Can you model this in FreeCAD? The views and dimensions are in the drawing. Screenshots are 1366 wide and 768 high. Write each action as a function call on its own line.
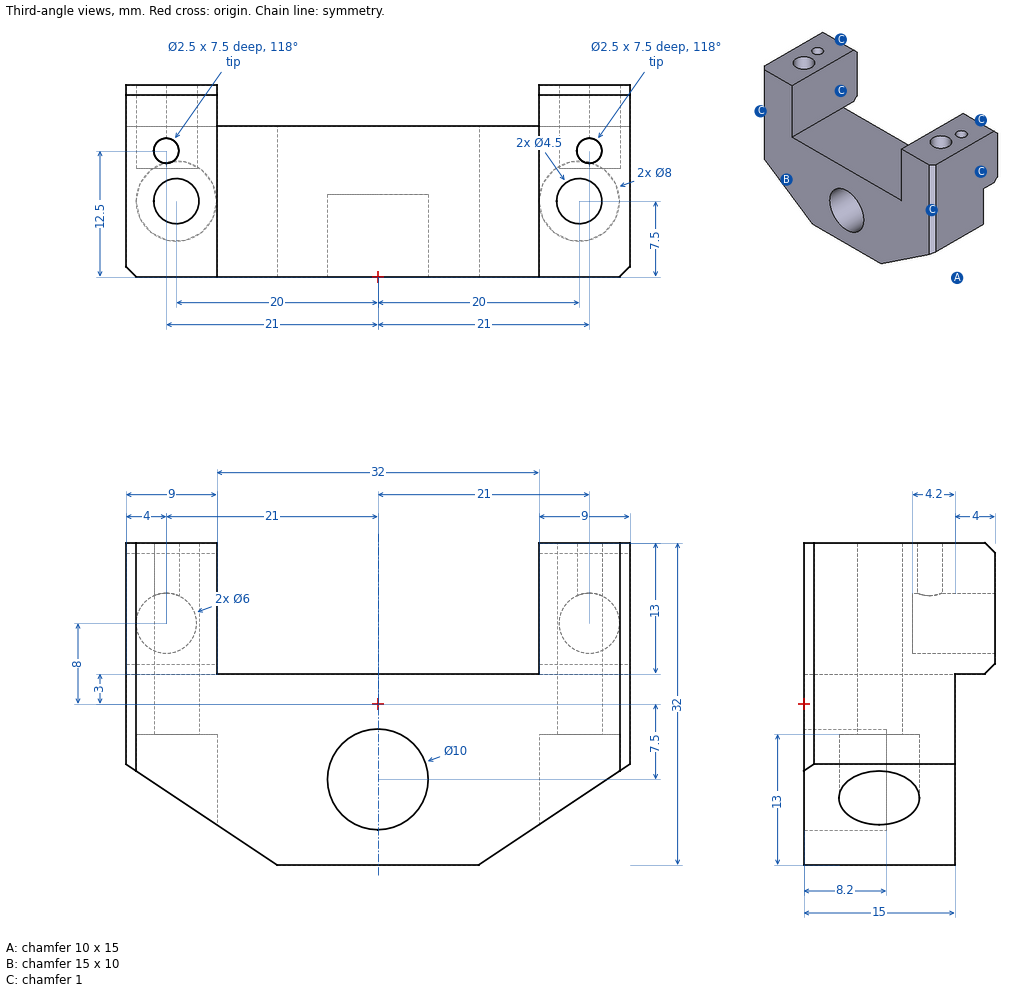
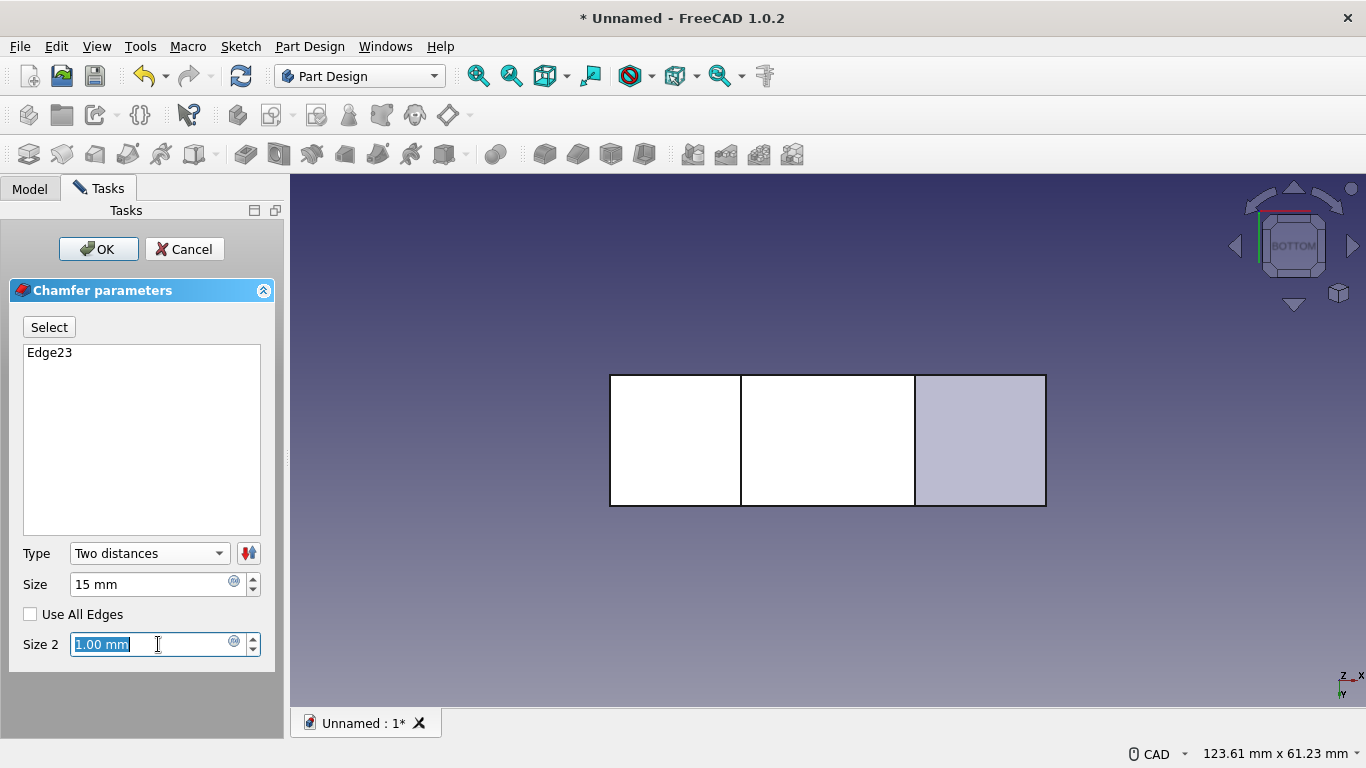
text(10)
key(Tab)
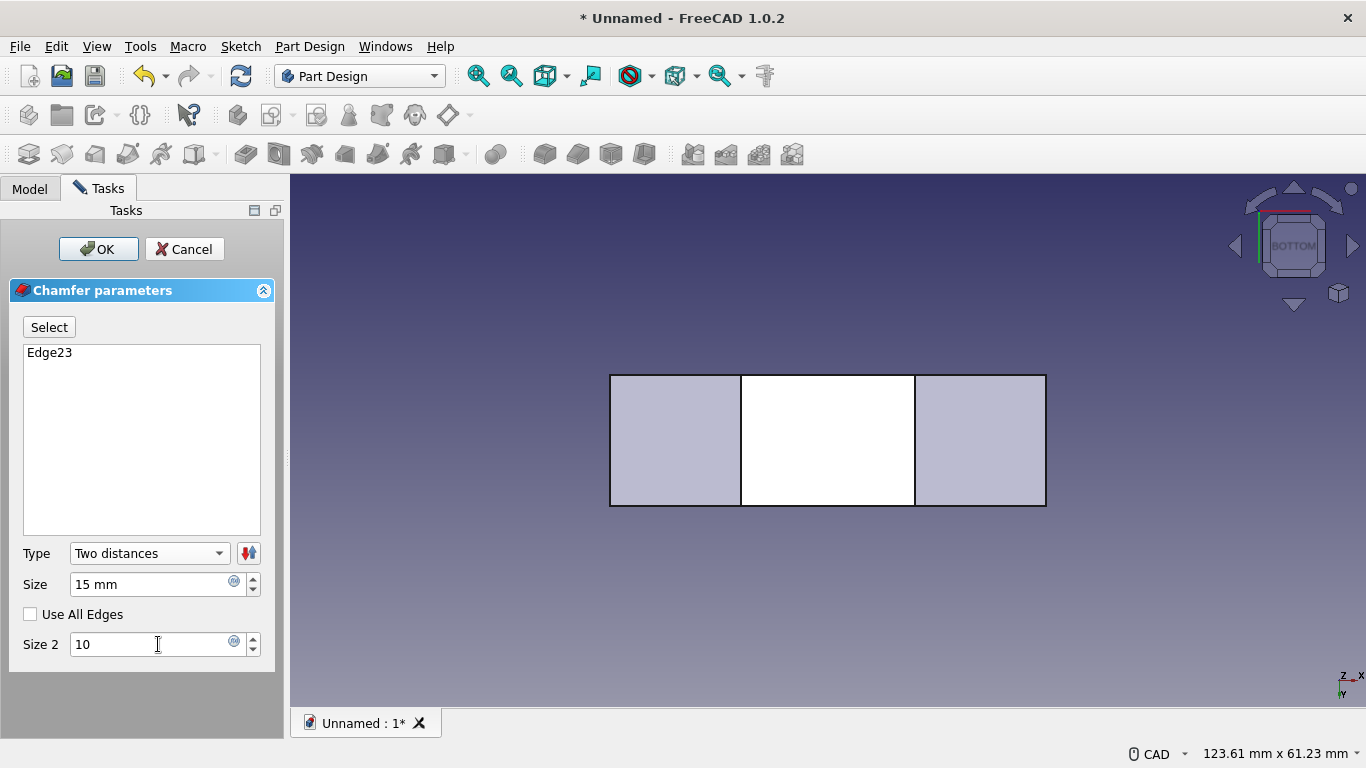
click(99, 249)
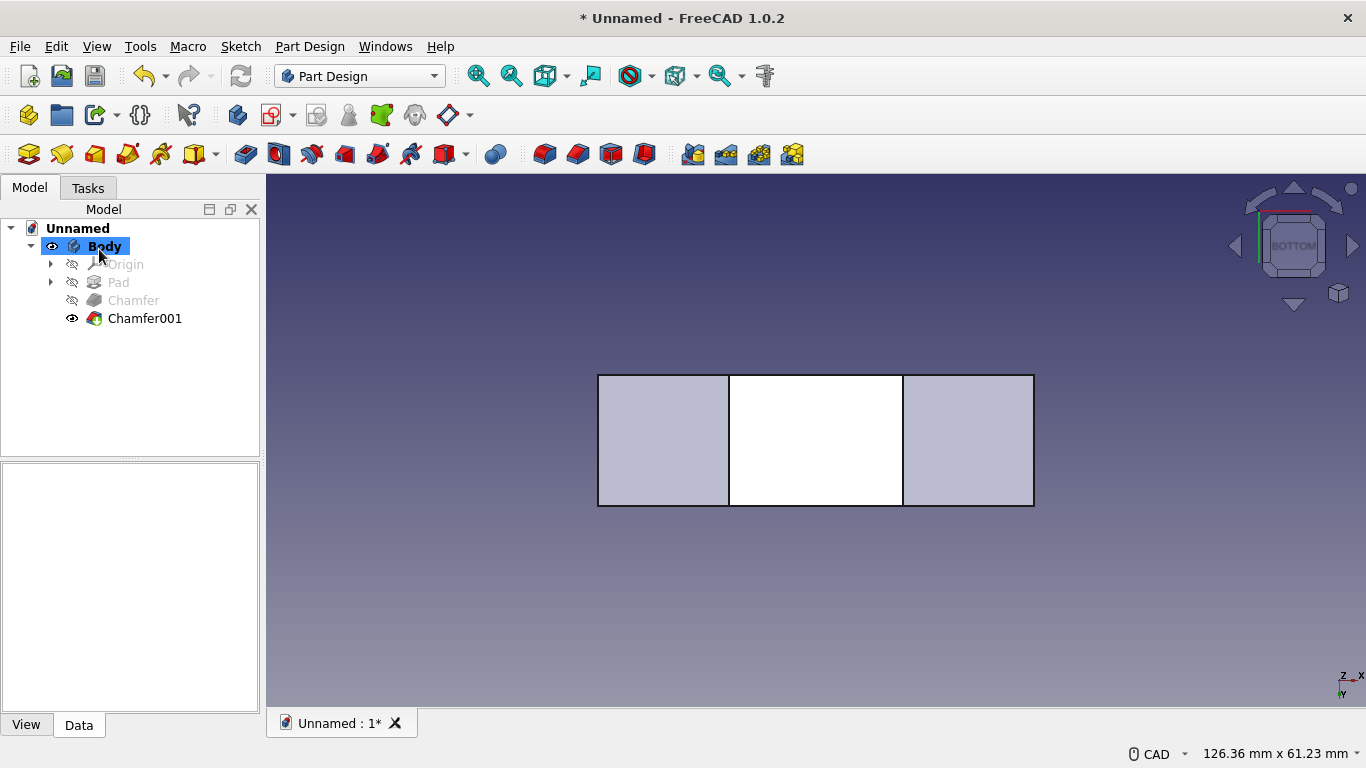
key(v)
key(f)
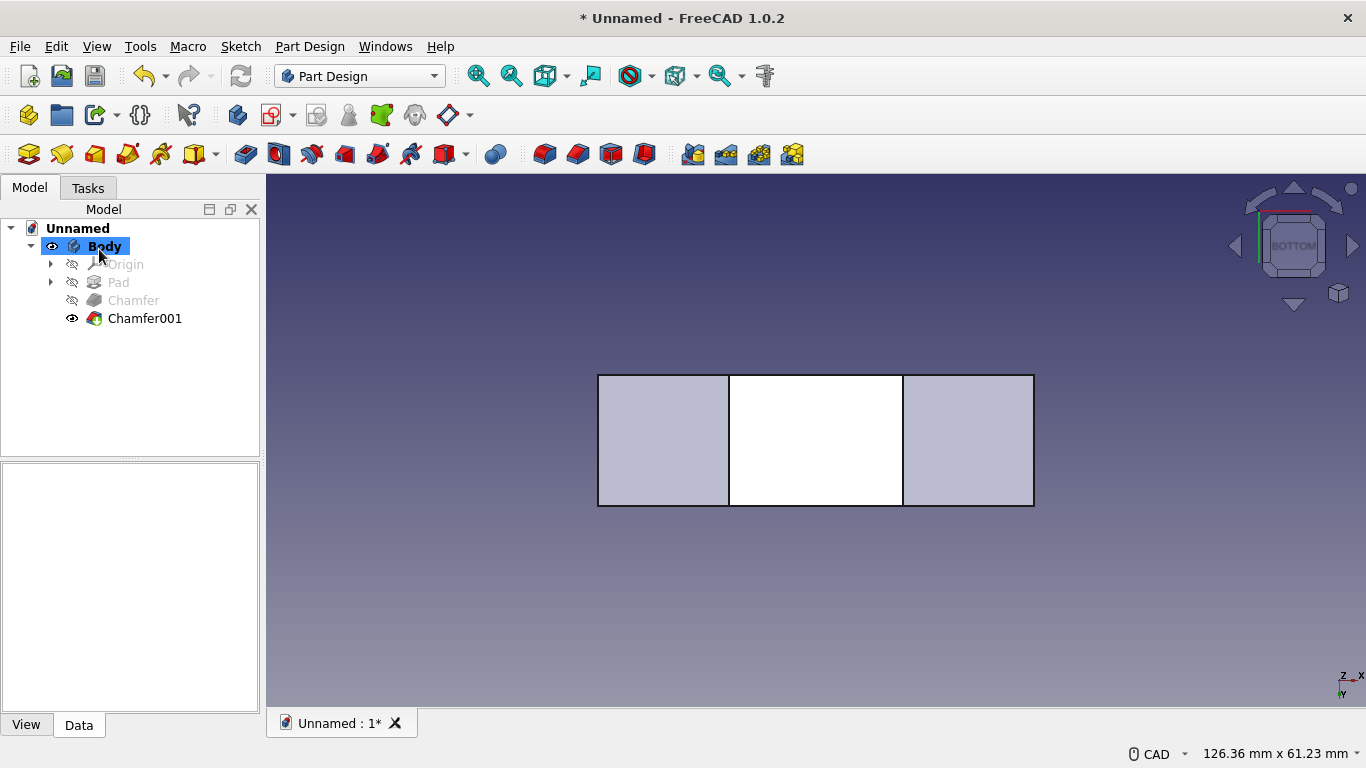
click(816, 439)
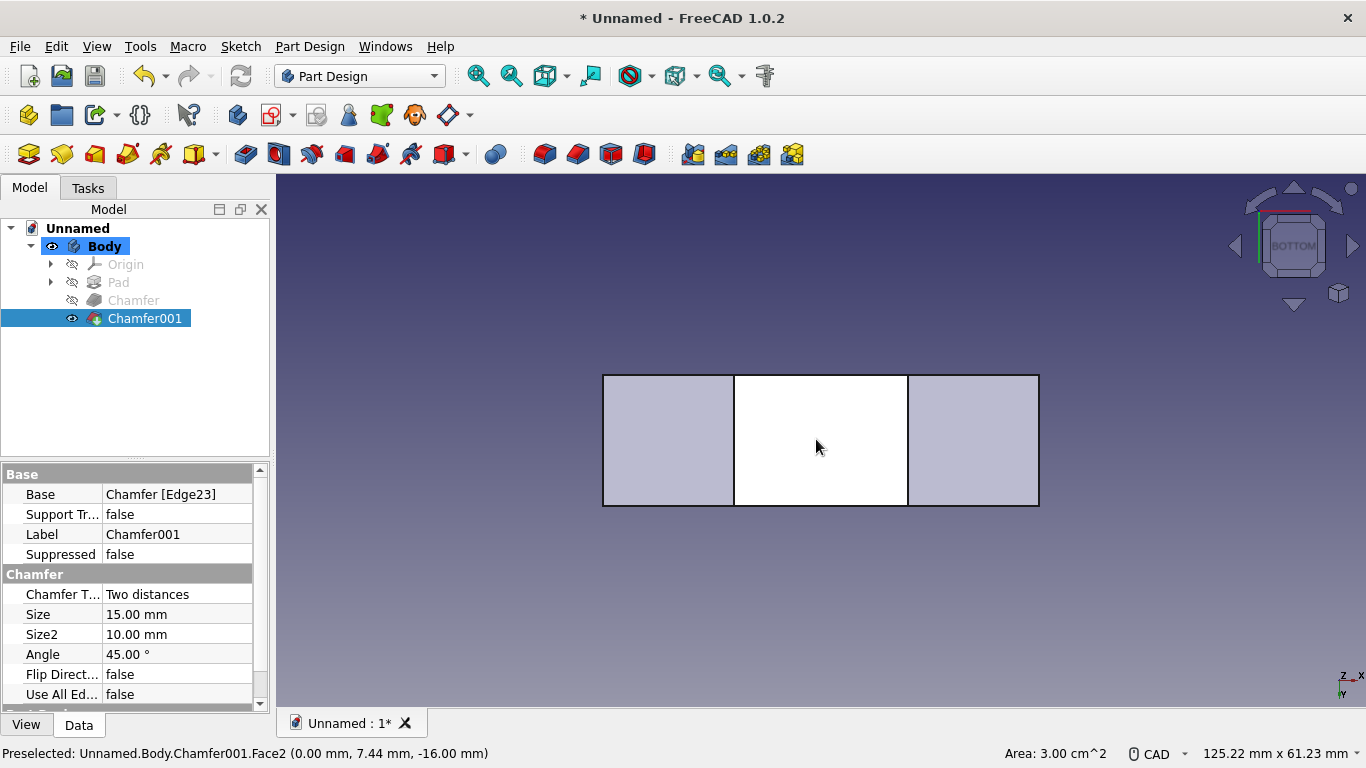
click(270, 116)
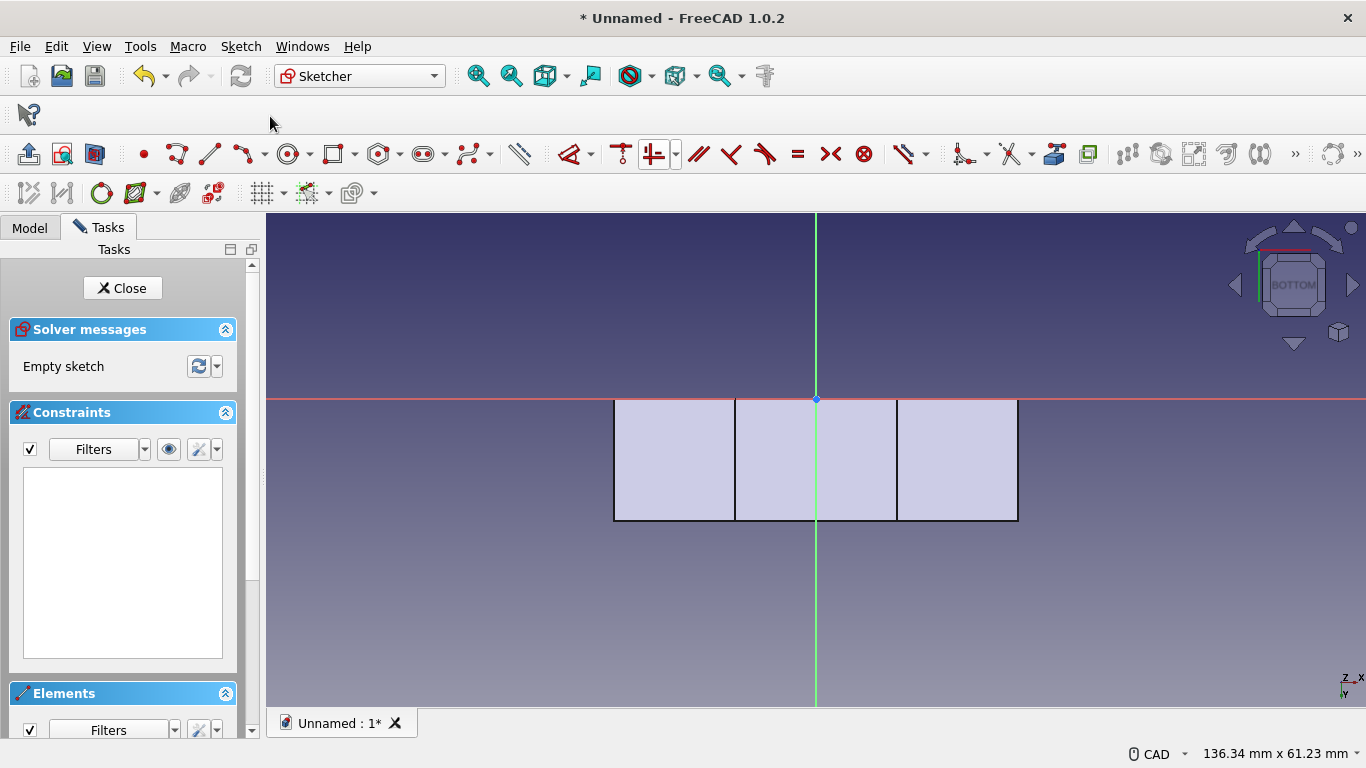
scroll(899, 413, up, 3)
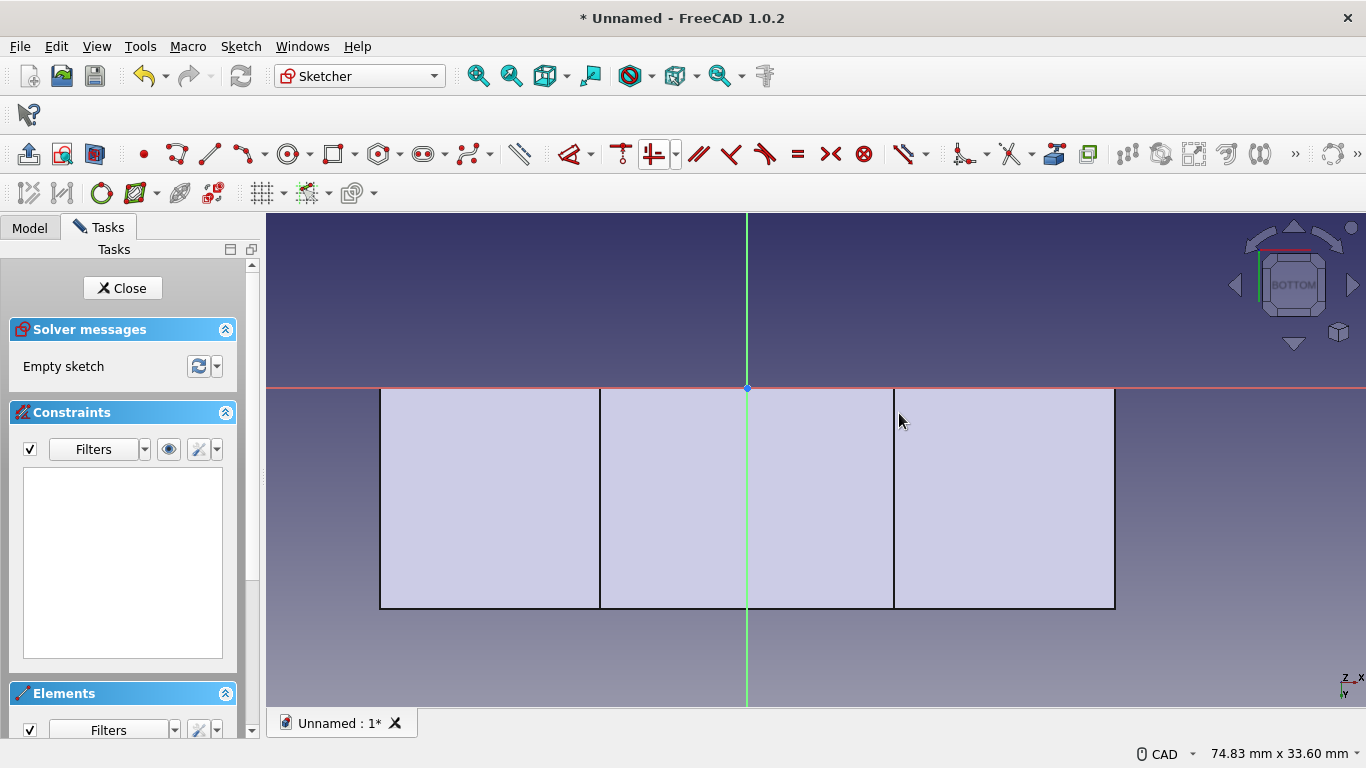
click(288, 154)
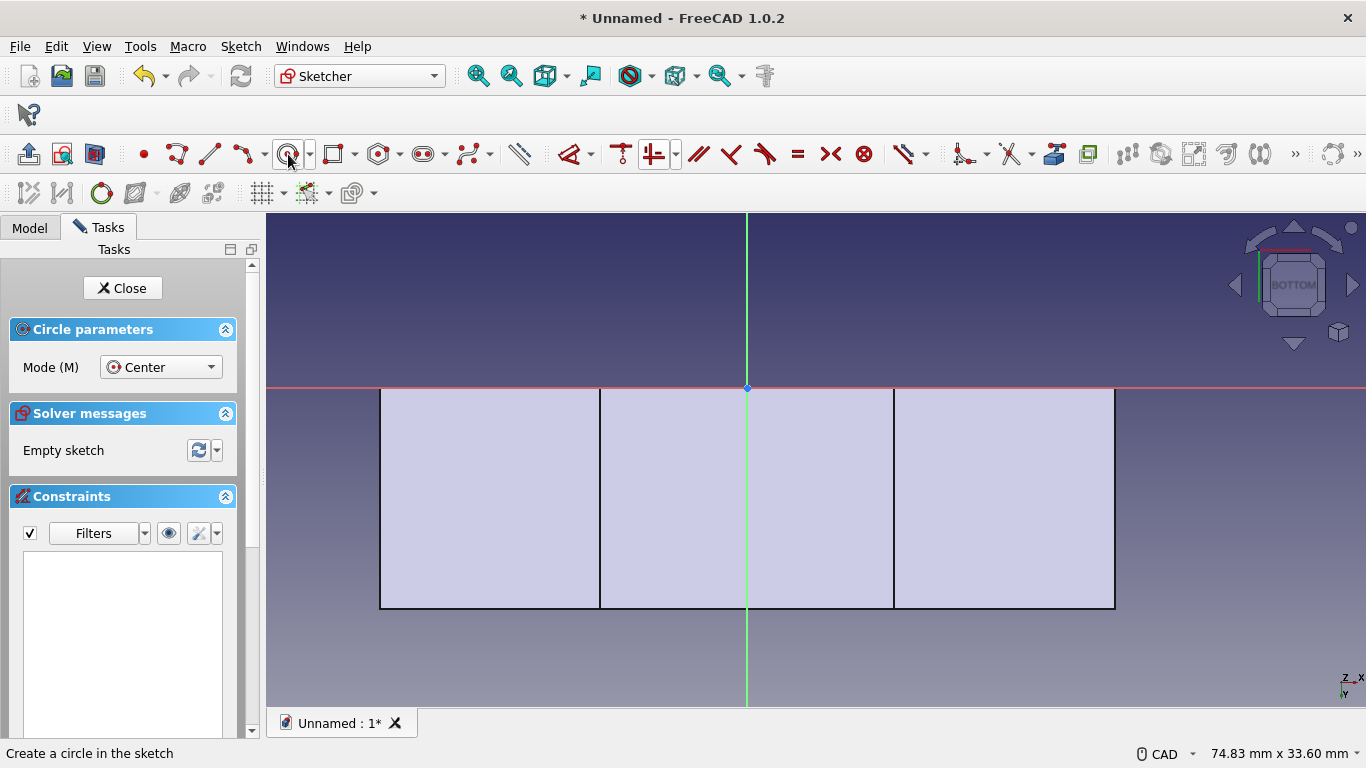
click(1041, 498)
move(1065, 475)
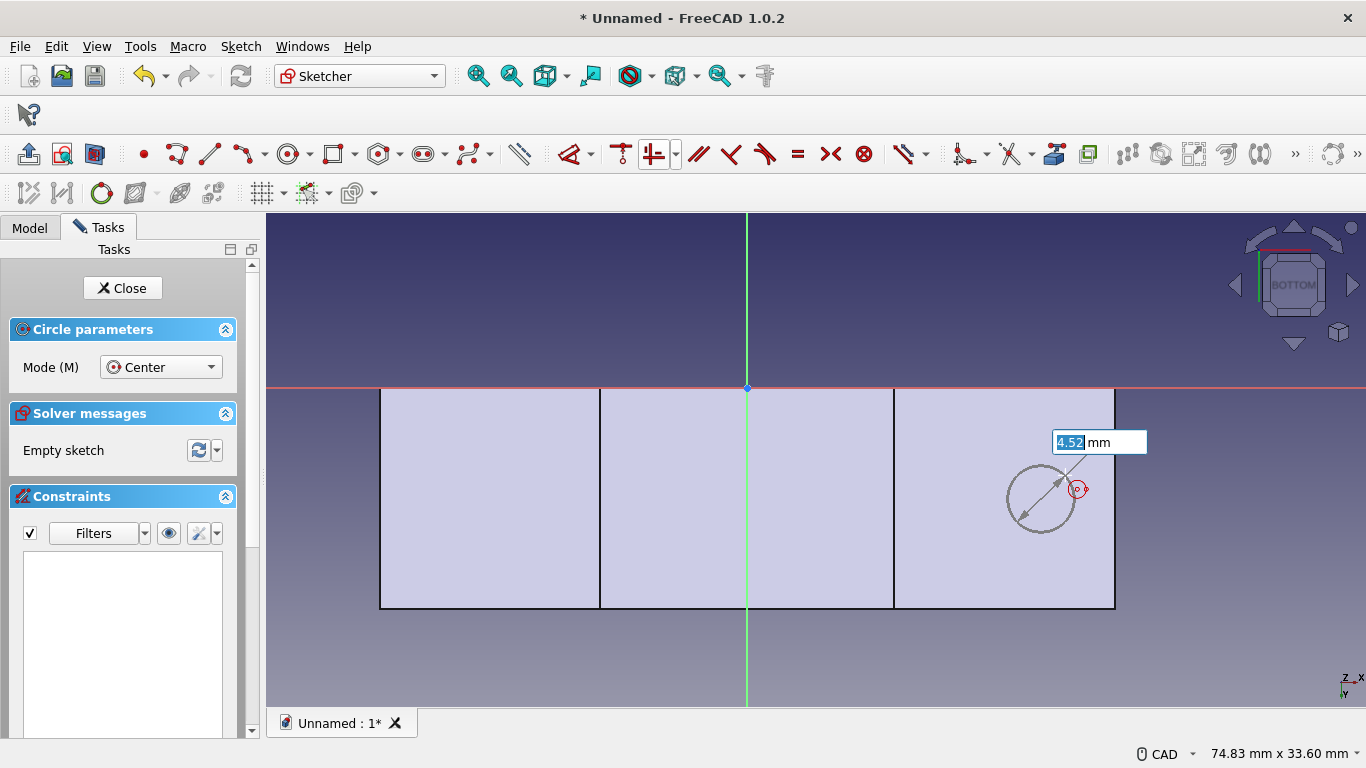
text(4.5)
key(Return)